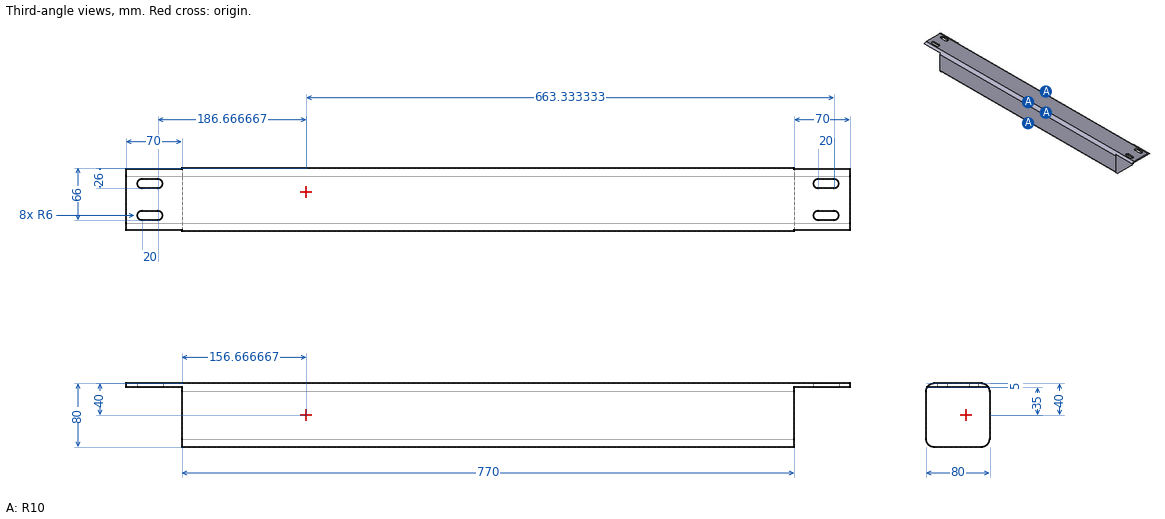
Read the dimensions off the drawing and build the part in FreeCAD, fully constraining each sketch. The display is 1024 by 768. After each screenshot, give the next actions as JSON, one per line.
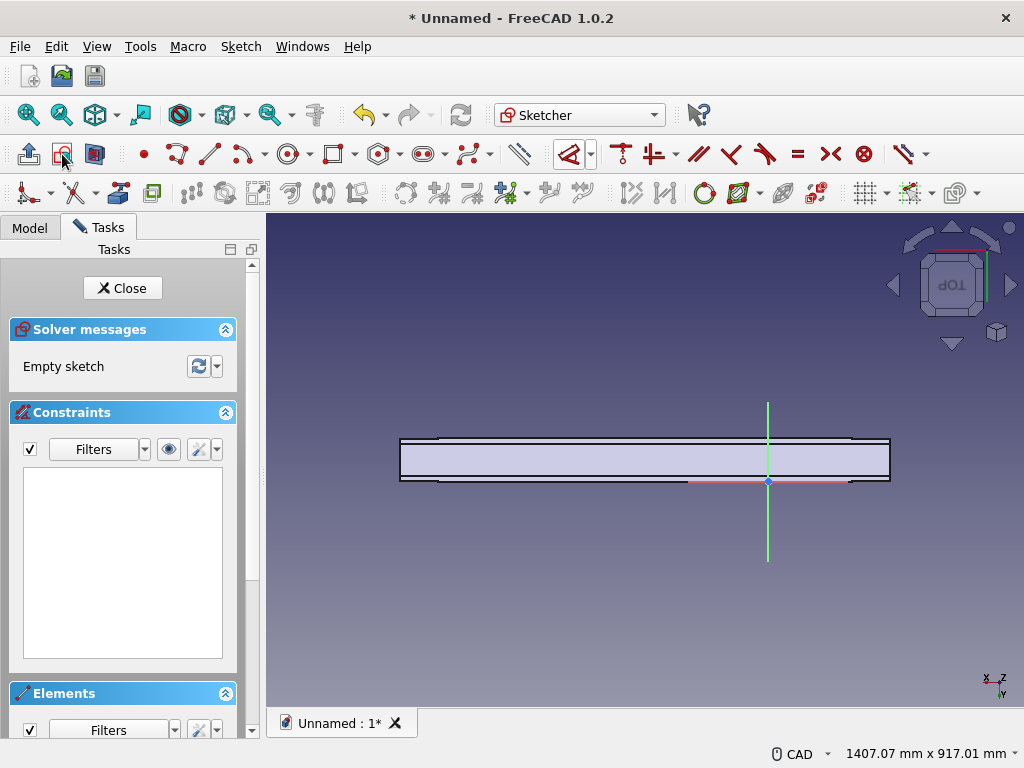
{"action": "scroll", "coordinate": [294, 443], "scroll_direction": "down", "scroll_amount": 1}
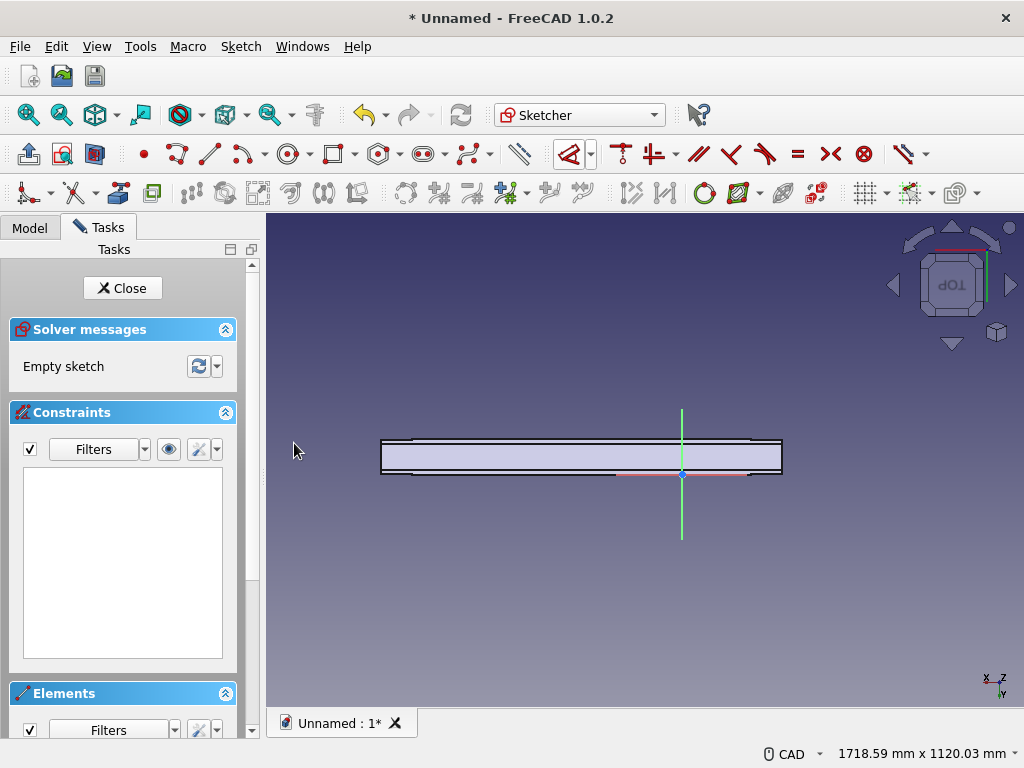
{"action": "left_click", "coordinate": [422, 154]}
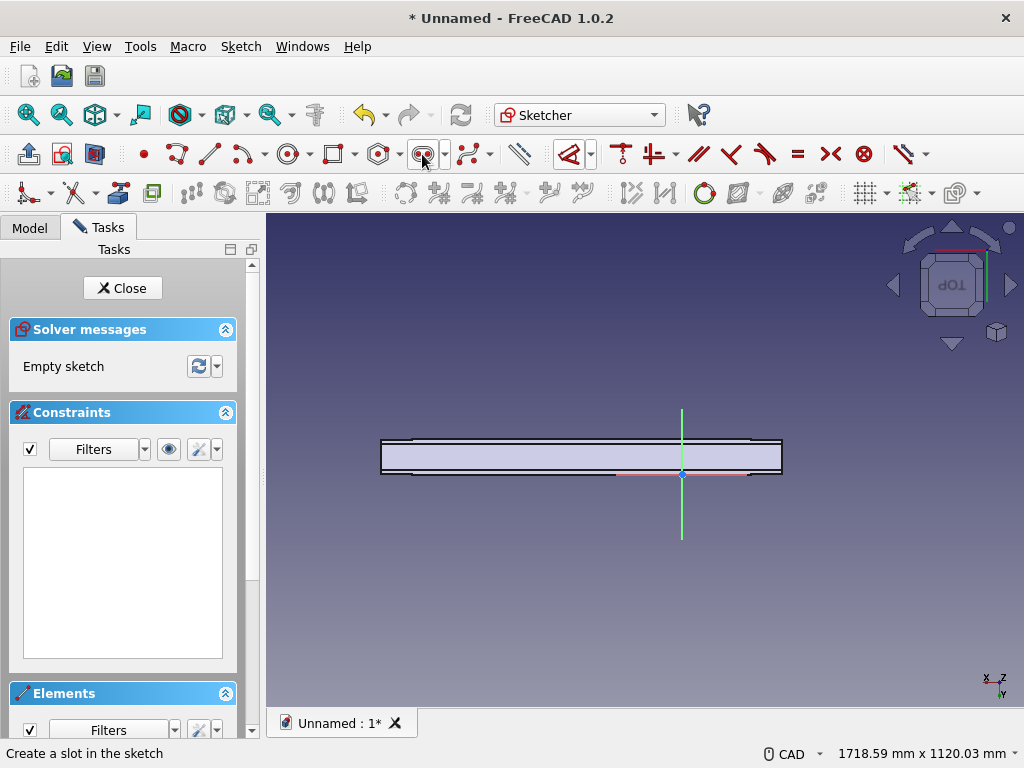
{"action": "scroll", "coordinate": [764, 448], "scroll_direction": "up", "scroll_amount": 11}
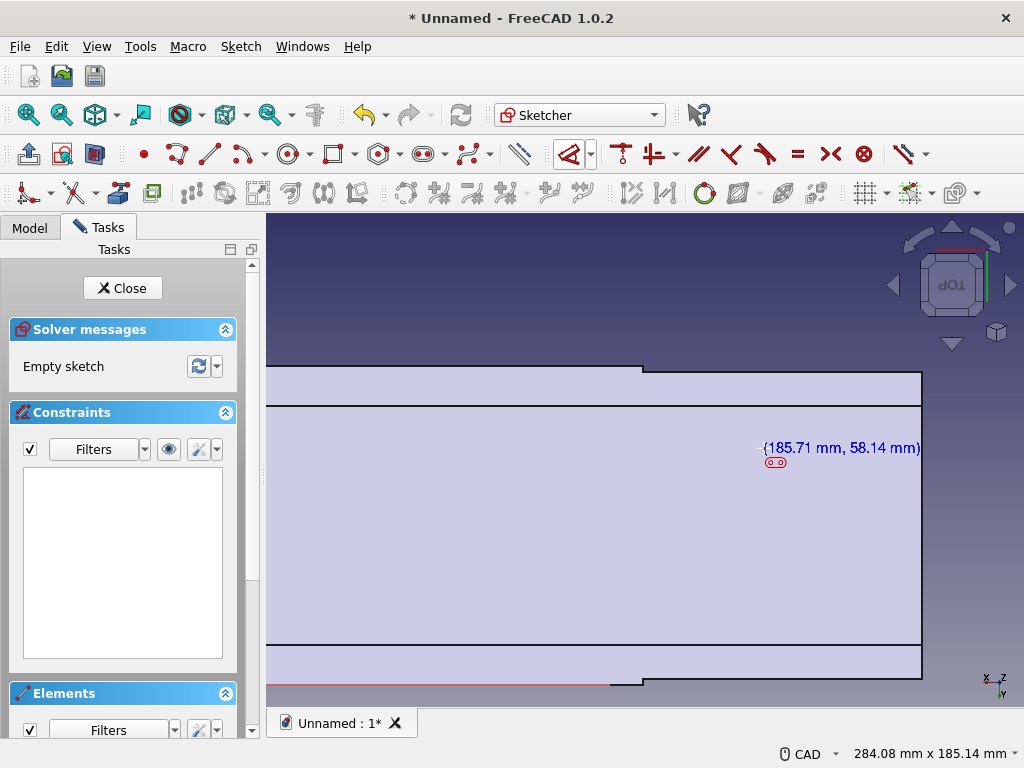
{"action": "scroll", "coordinate": [759, 448], "scroll_direction": "down", "scroll_amount": 11}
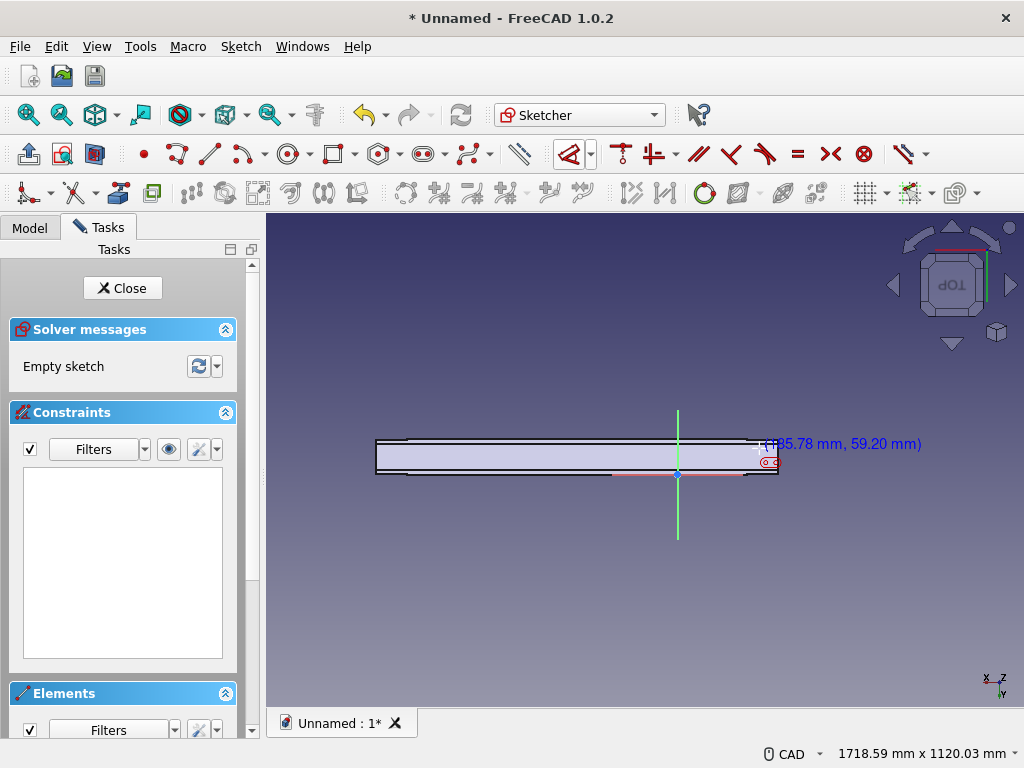
{"action": "left_click", "coordinate": [760, 448]}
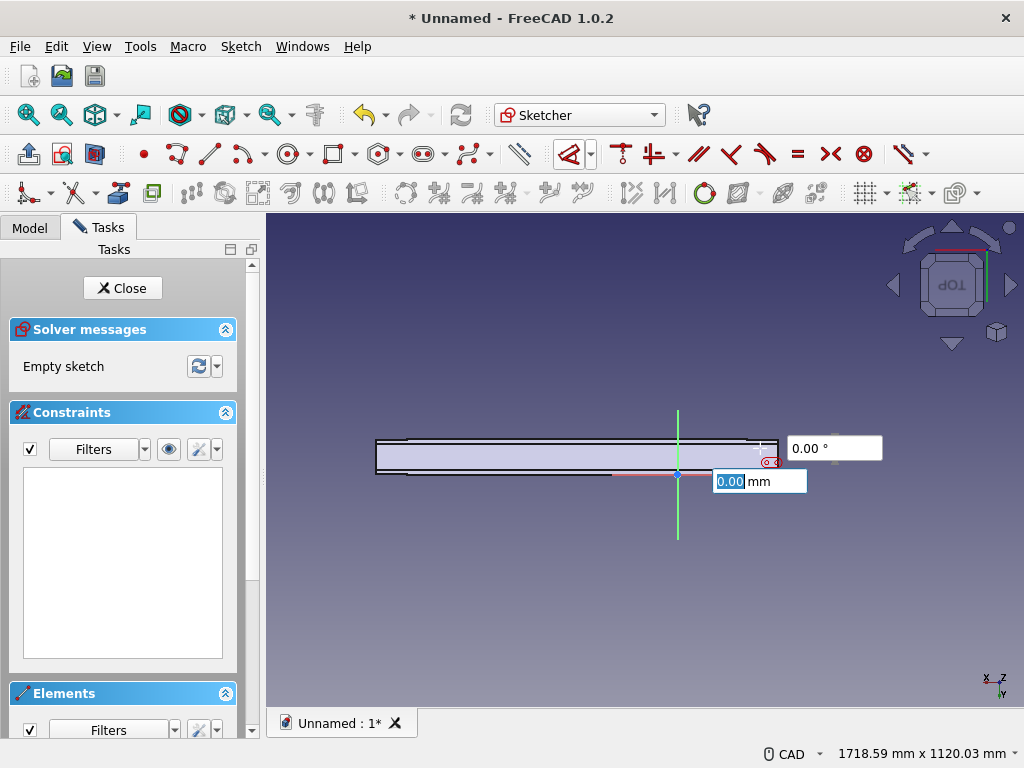
{"action": "scroll", "coordinate": [769, 448], "scroll_direction": "up", "scroll_amount": 3}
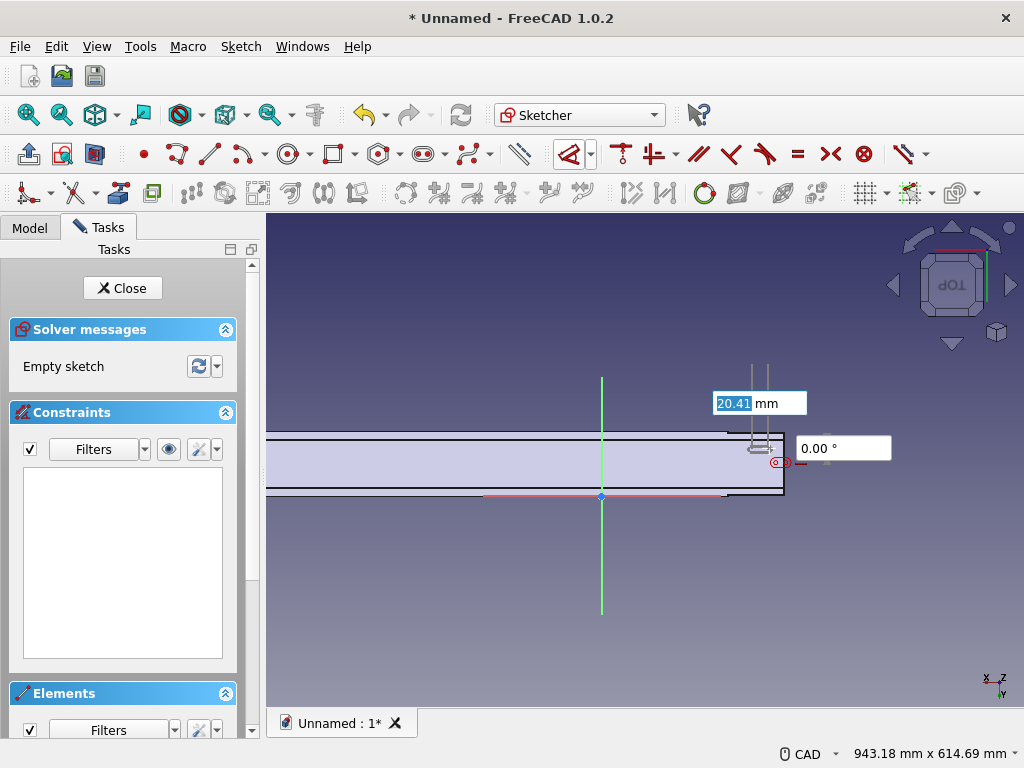
{"action": "left_click", "coordinate": [768, 448]}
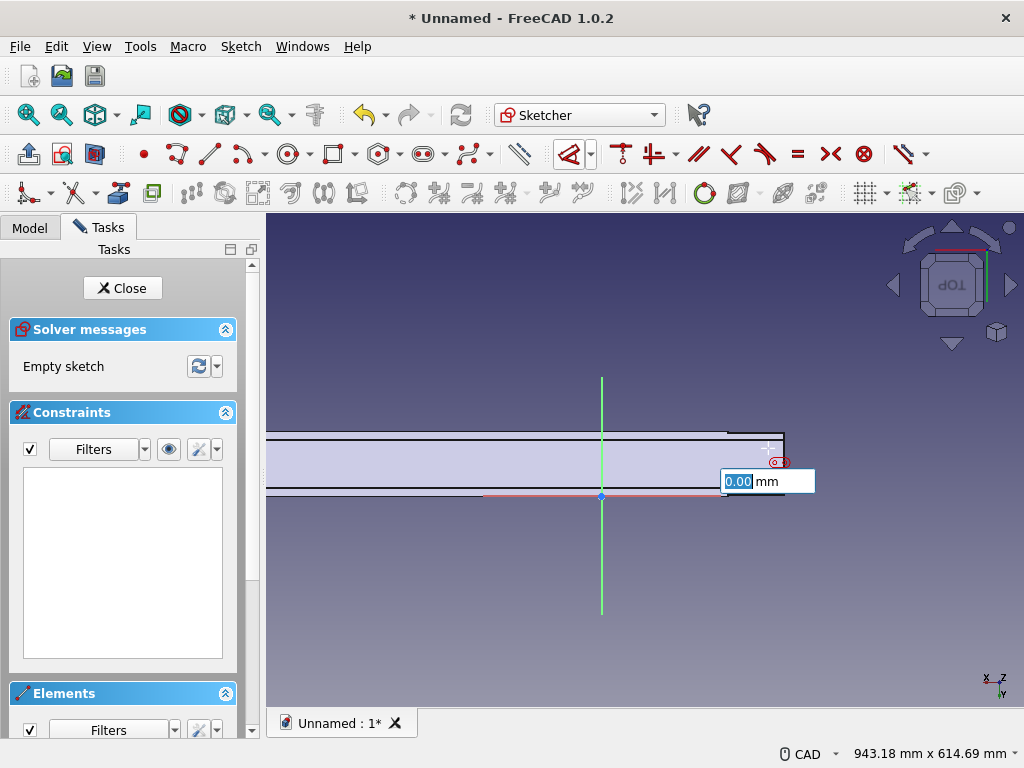
{"action": "scroll", "coordinate": [760, 453], "scroll_direction": "up", "scroll_amount": 6}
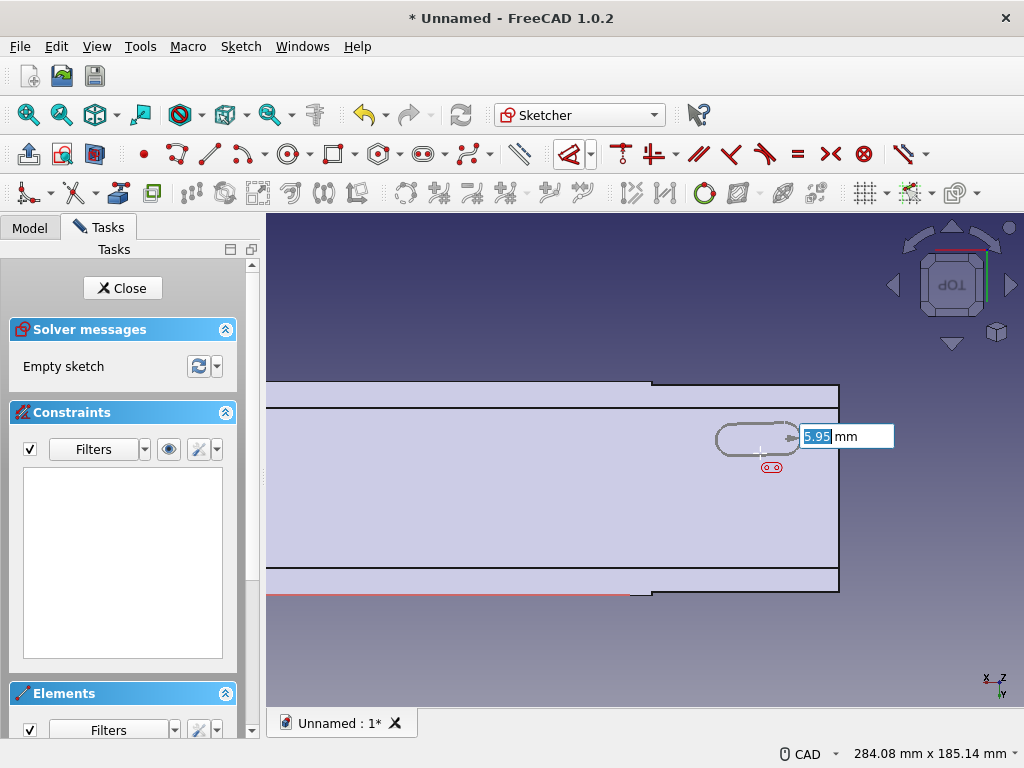
{"action": "left_click", "coordinate": [759, 451]}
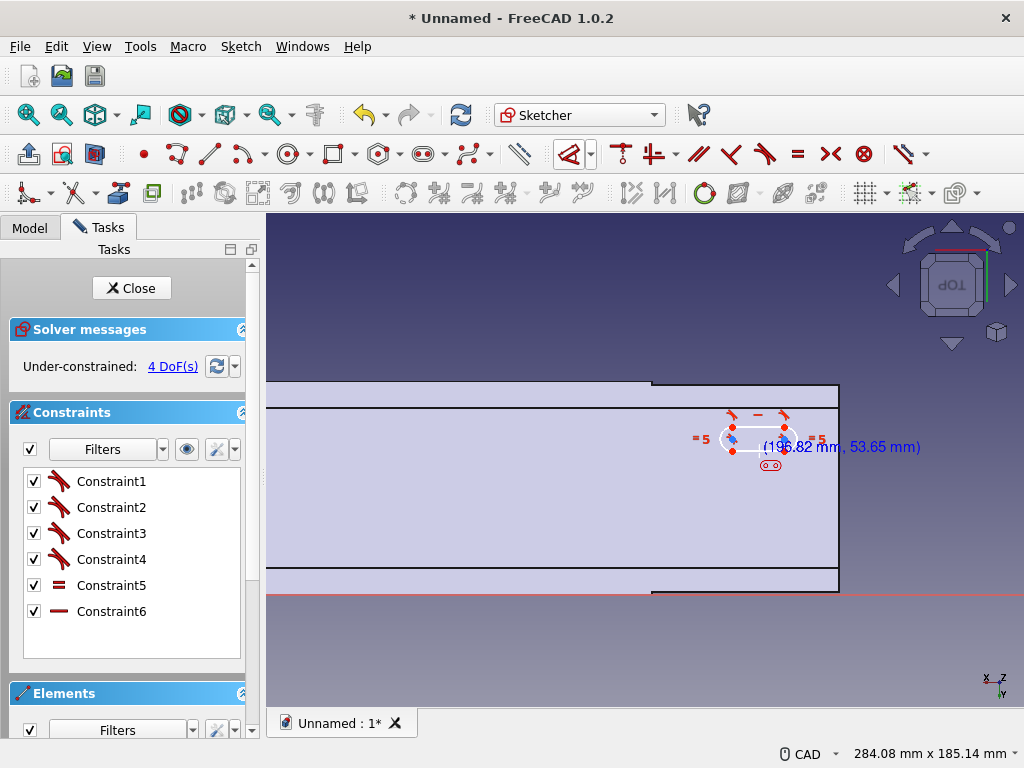
{"action": "scroll", "coordinate": [732, 542], "scroll_direction": "up", "scroll_amount": 2}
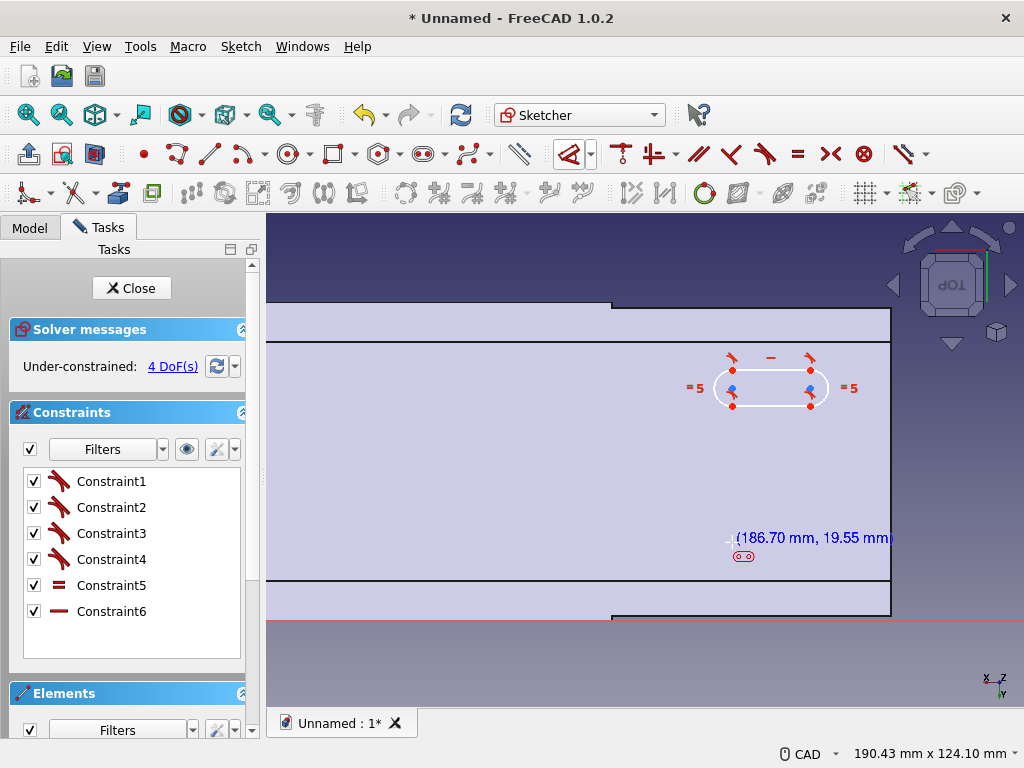
{"action": "scroll", "coordinate": [763, 456], "scroll_direction": "down", "scroll_amount": 11}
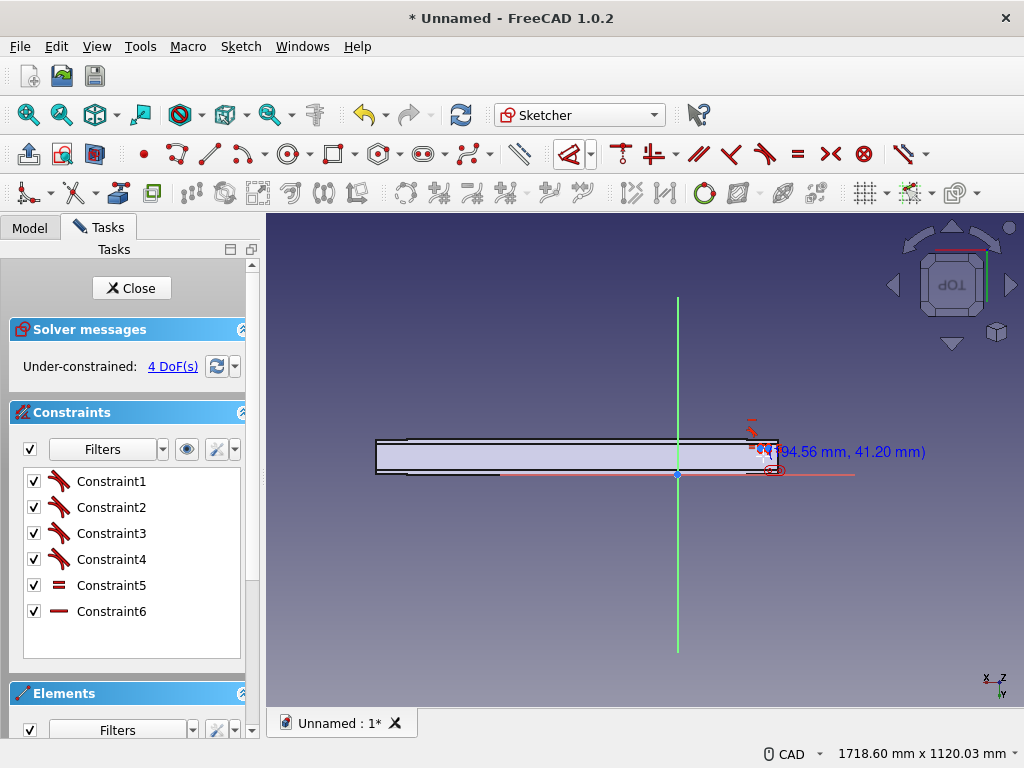
{"action": "scroll", "coordinate": [760, 466], "scroll_direction": "up", "scroll_amount": 3}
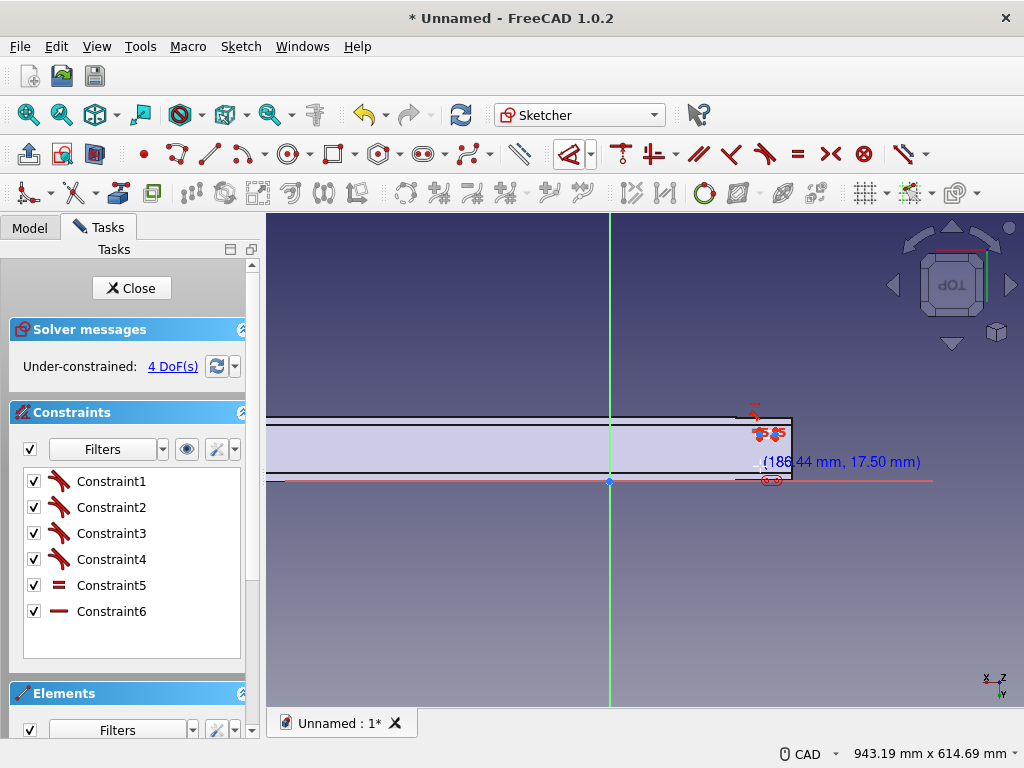
{"action": "left_click", "coordinate": [760, 465]}